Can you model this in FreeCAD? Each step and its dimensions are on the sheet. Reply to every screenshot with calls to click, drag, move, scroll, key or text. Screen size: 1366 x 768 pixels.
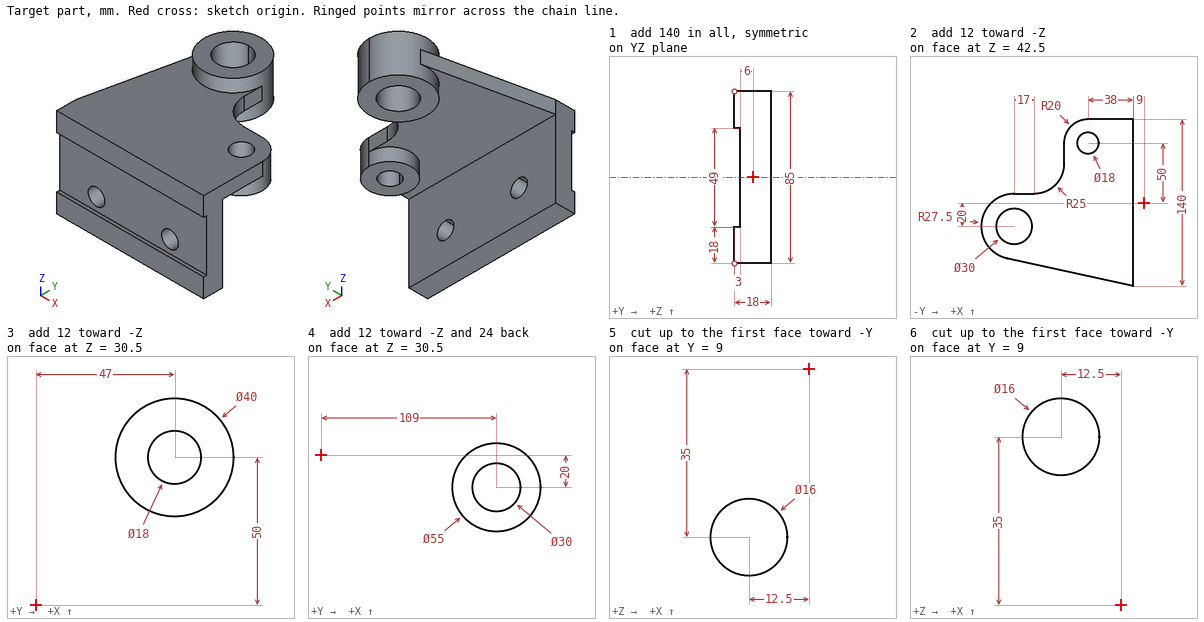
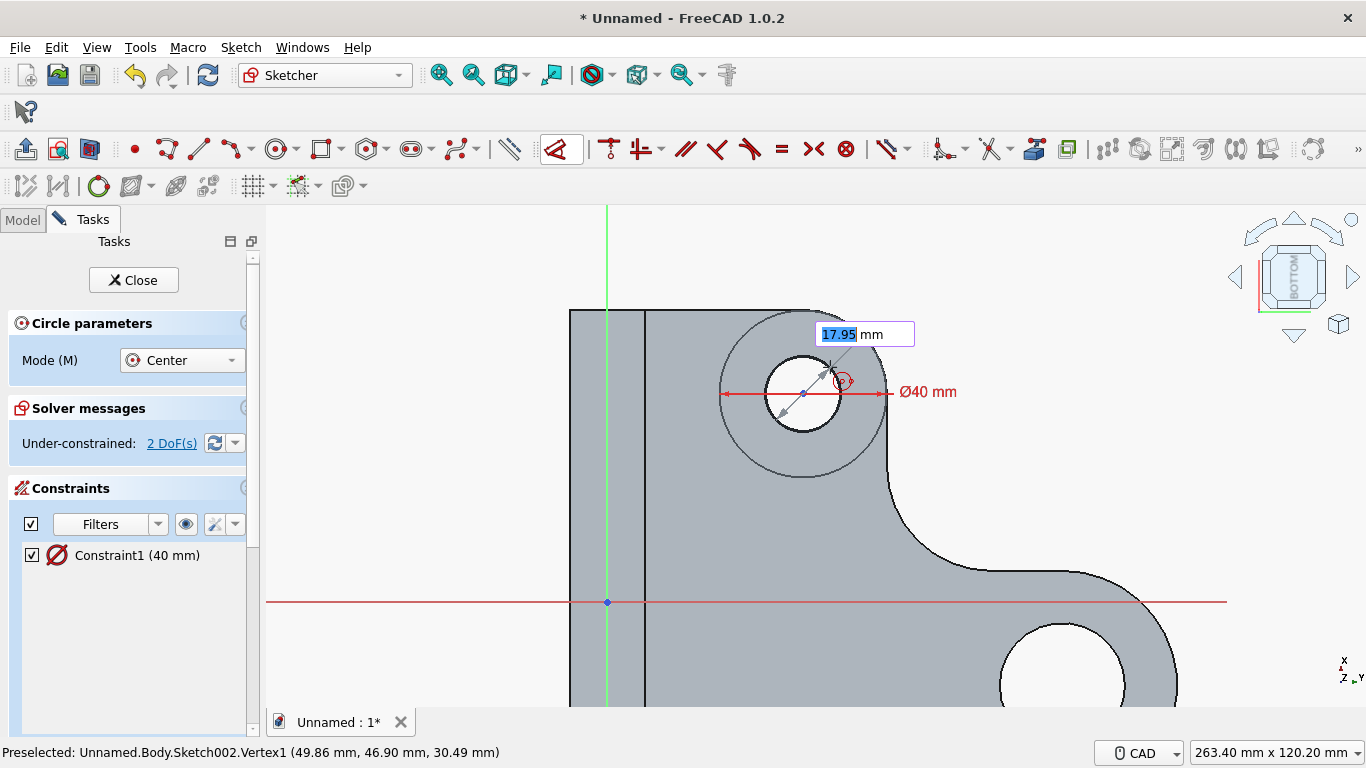
text(18)
key(Return)
key(Escape)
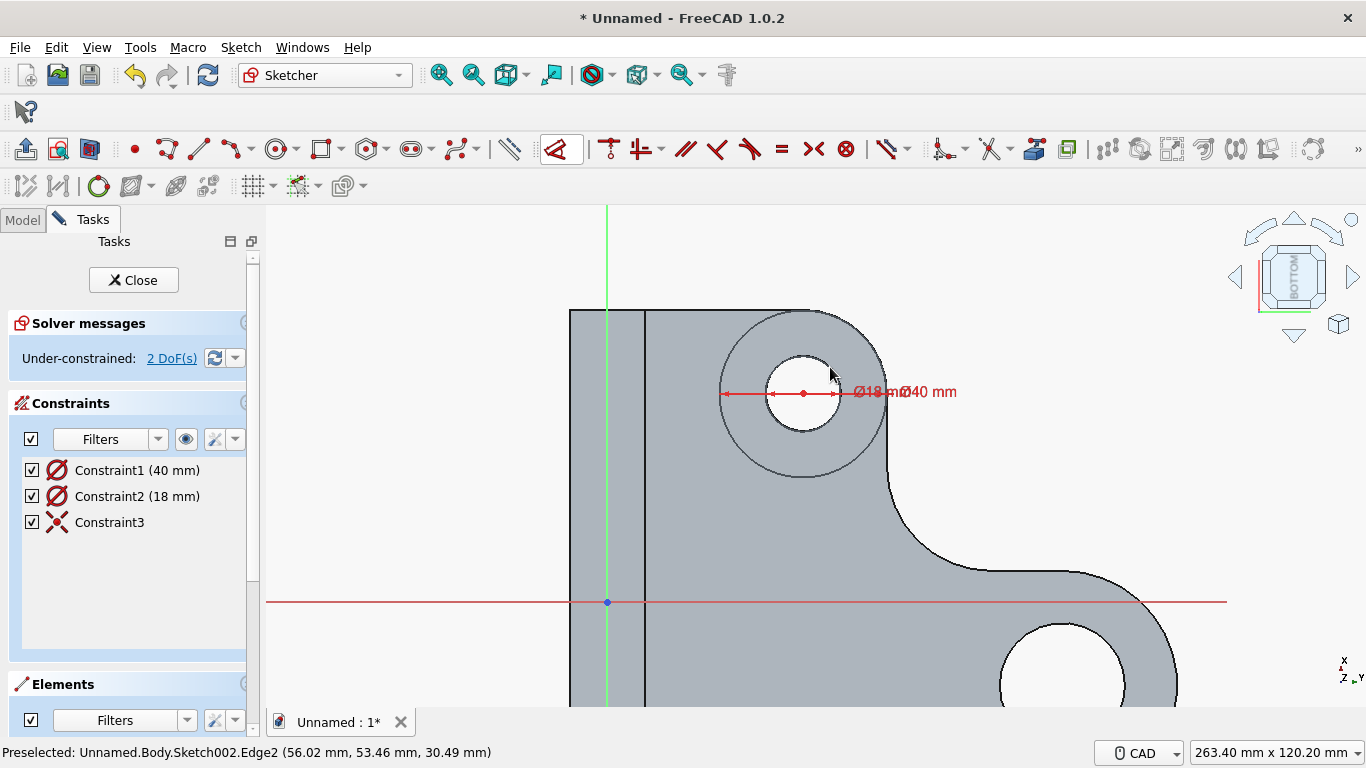
click(803, 394)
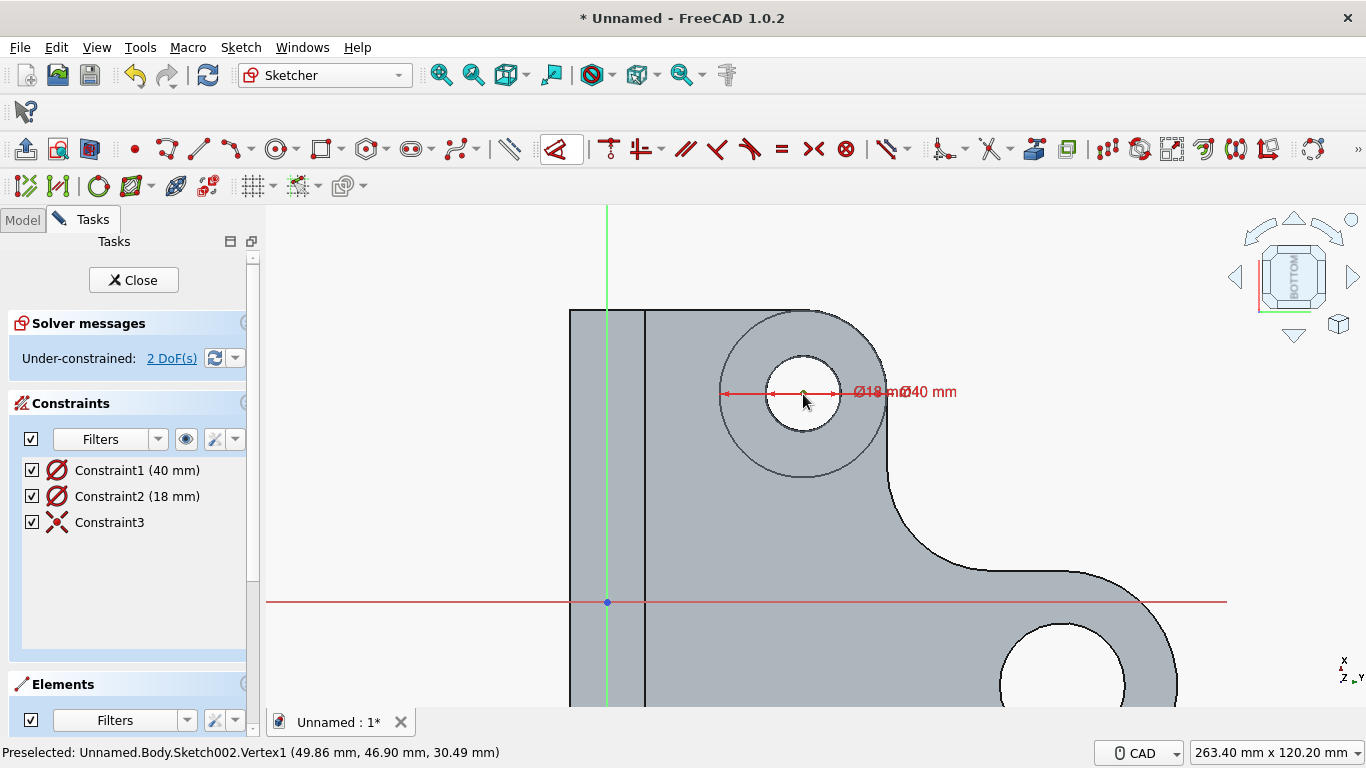
key(l)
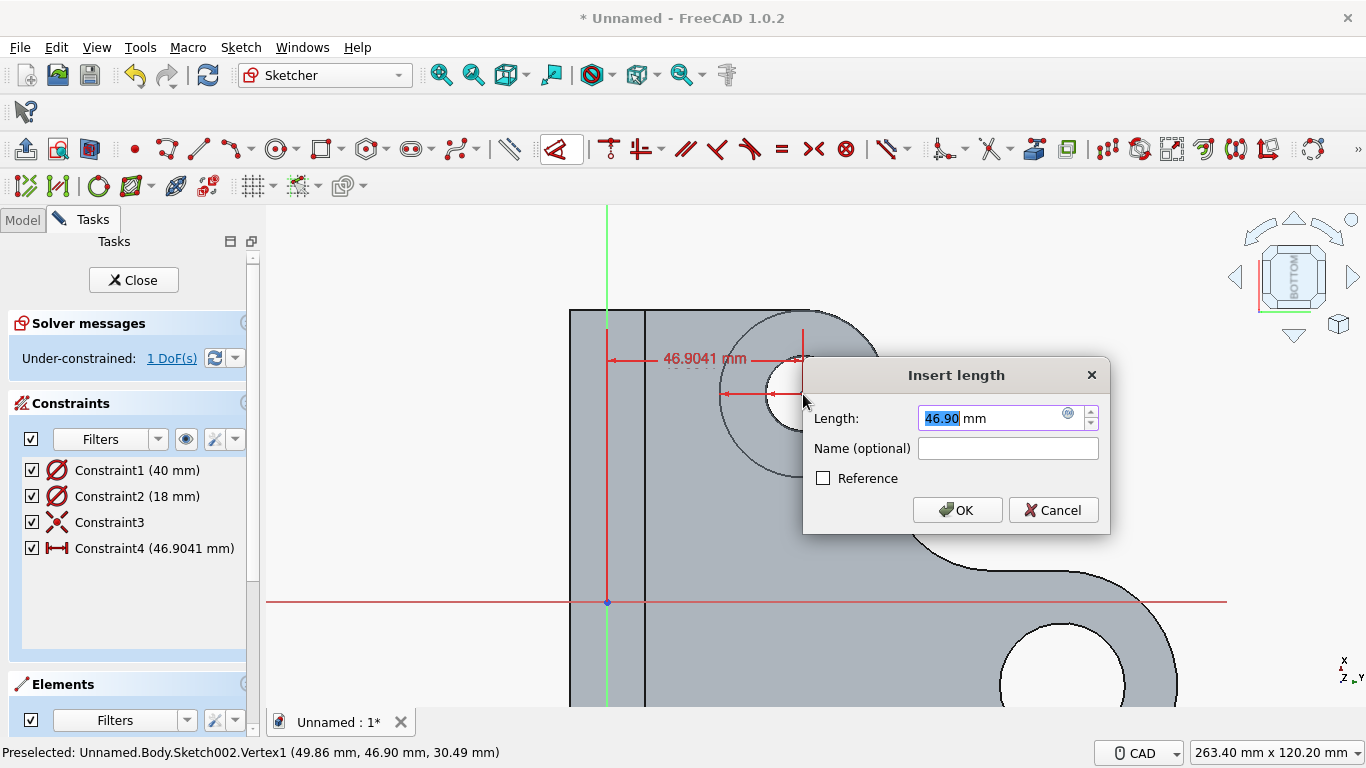
text(47)
key(Return)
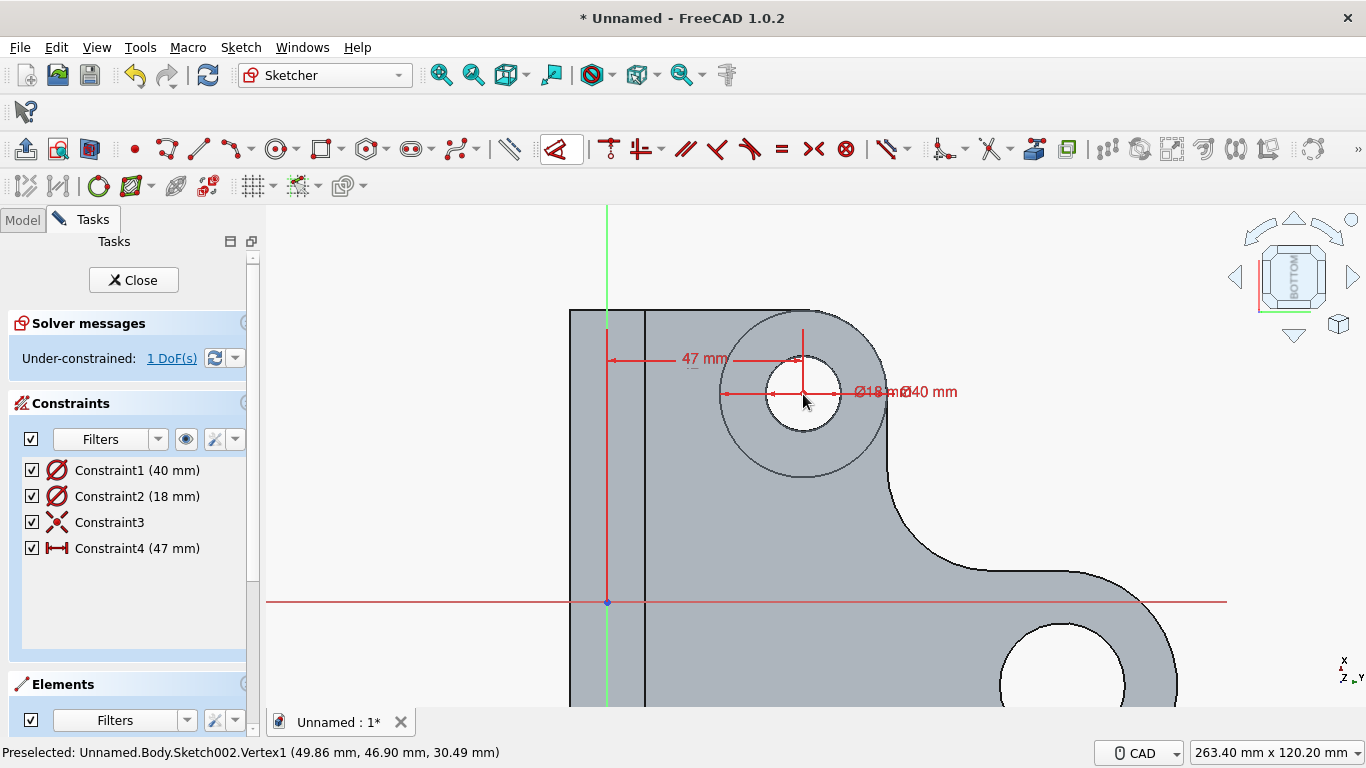
click(803, 394)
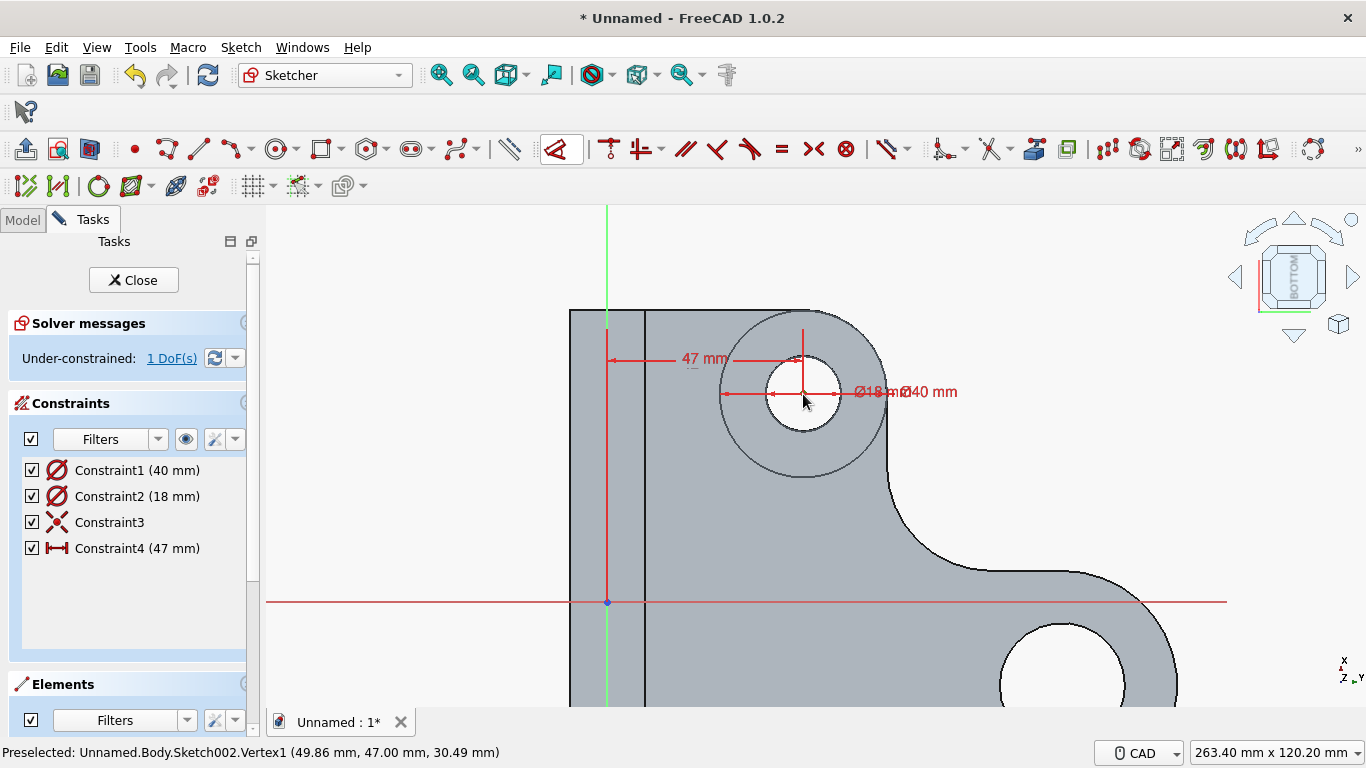
click(578, 150)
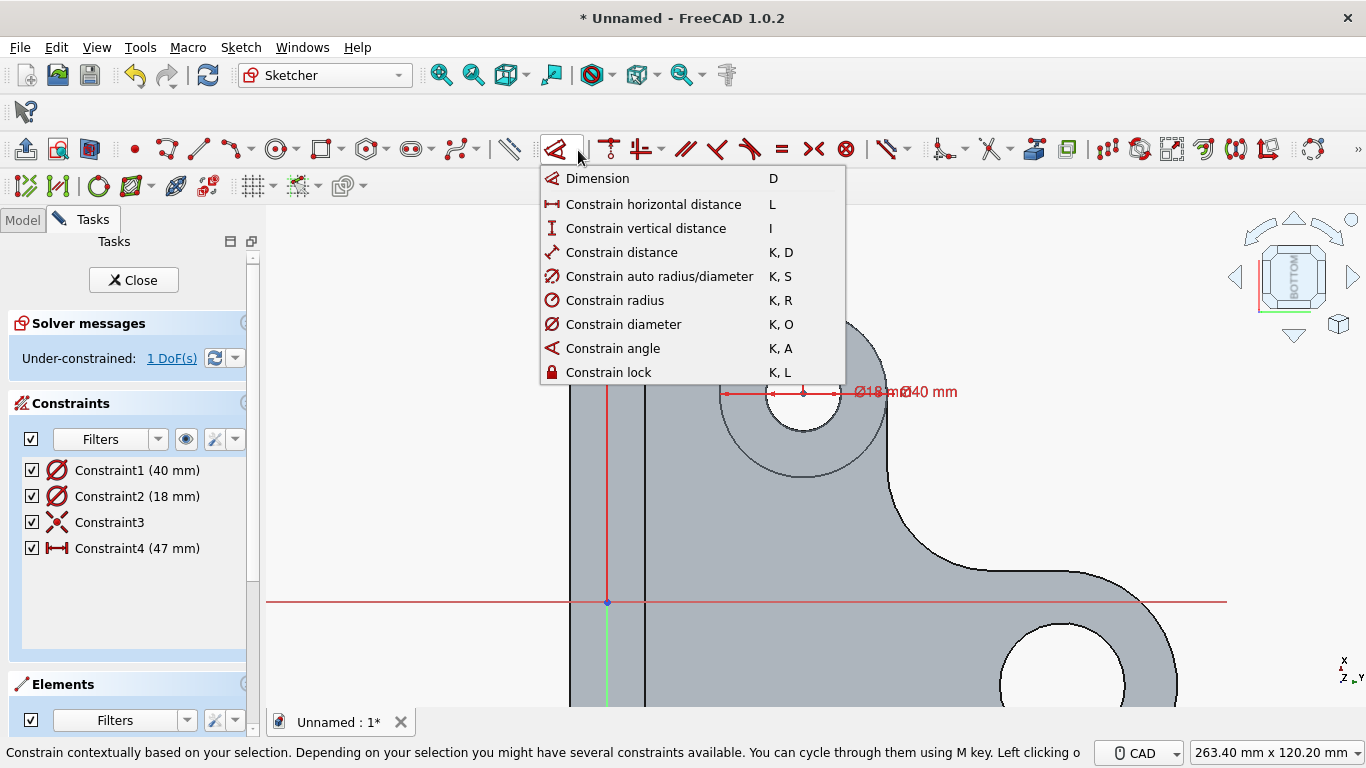
click(693, 228)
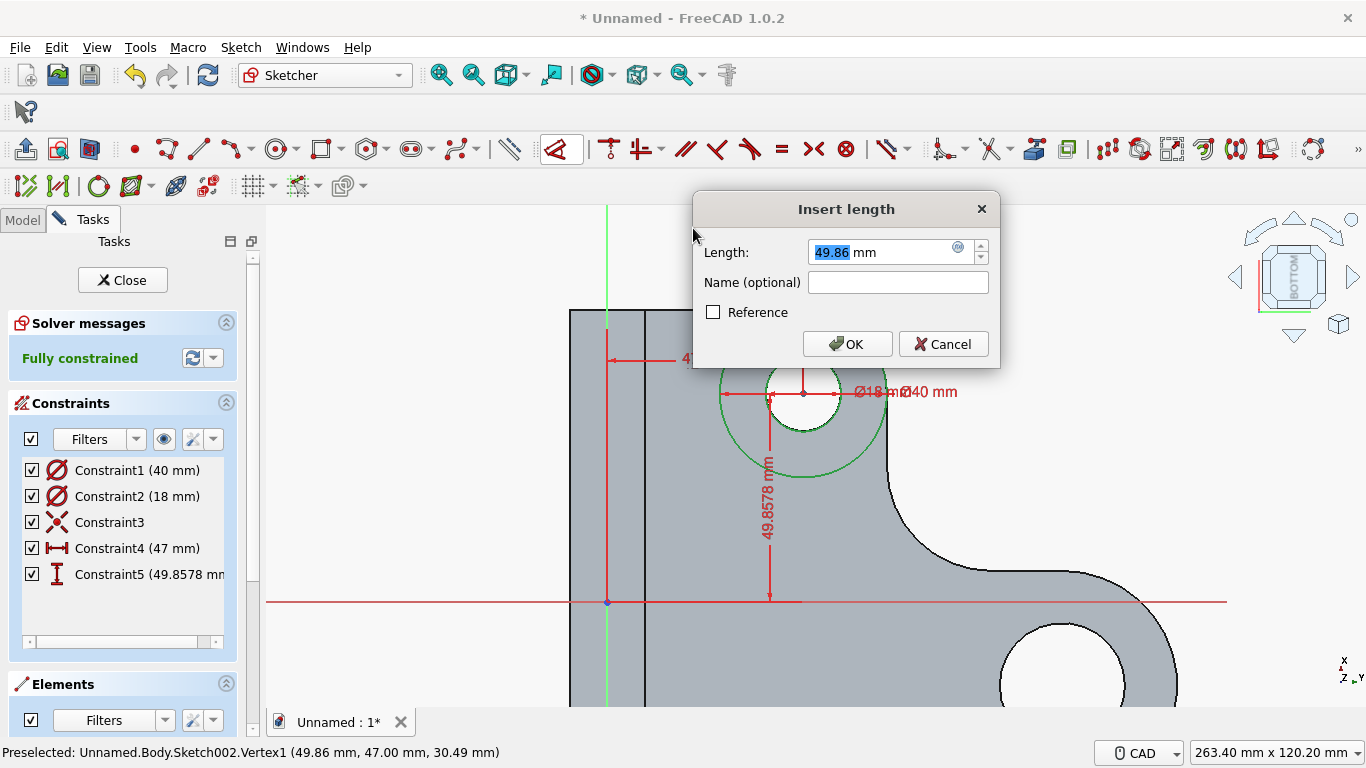
text(50)
key(Return)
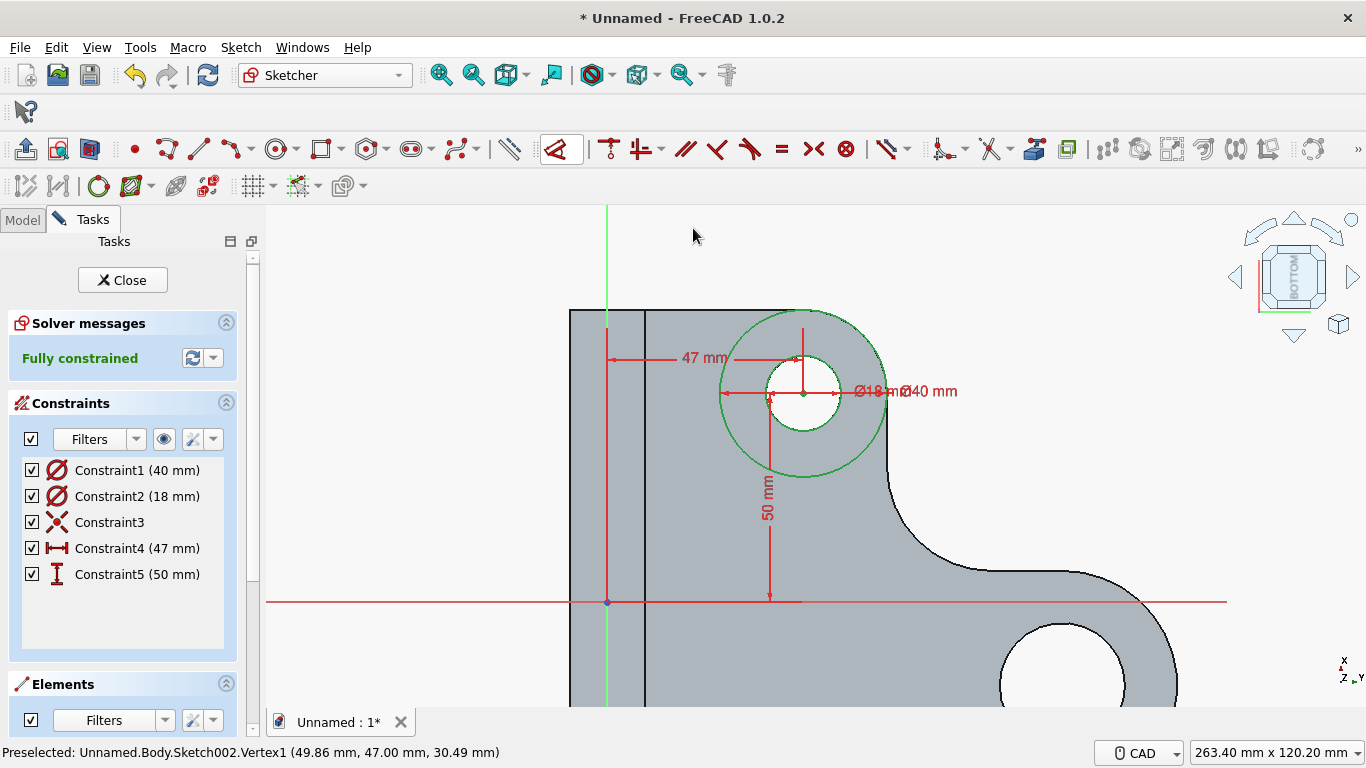
click(123, 280)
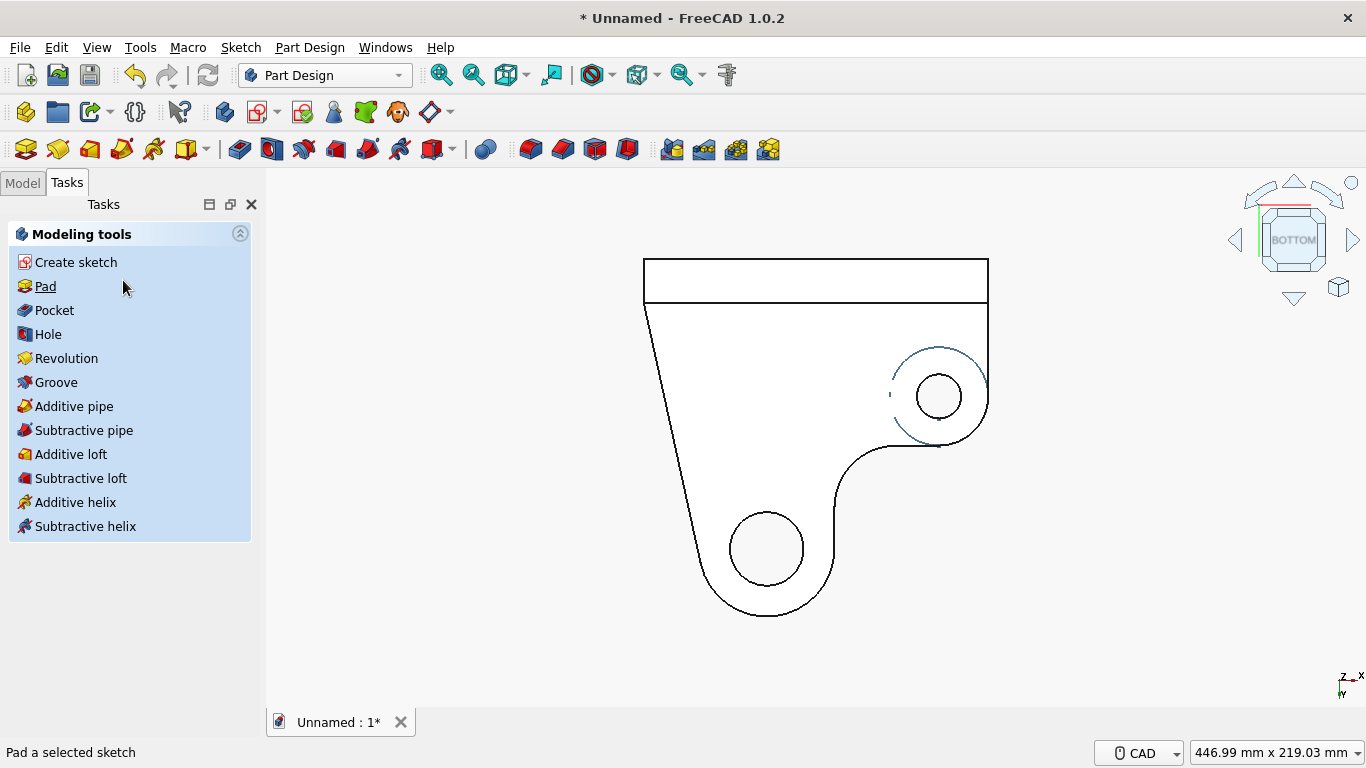
click(26, 150)